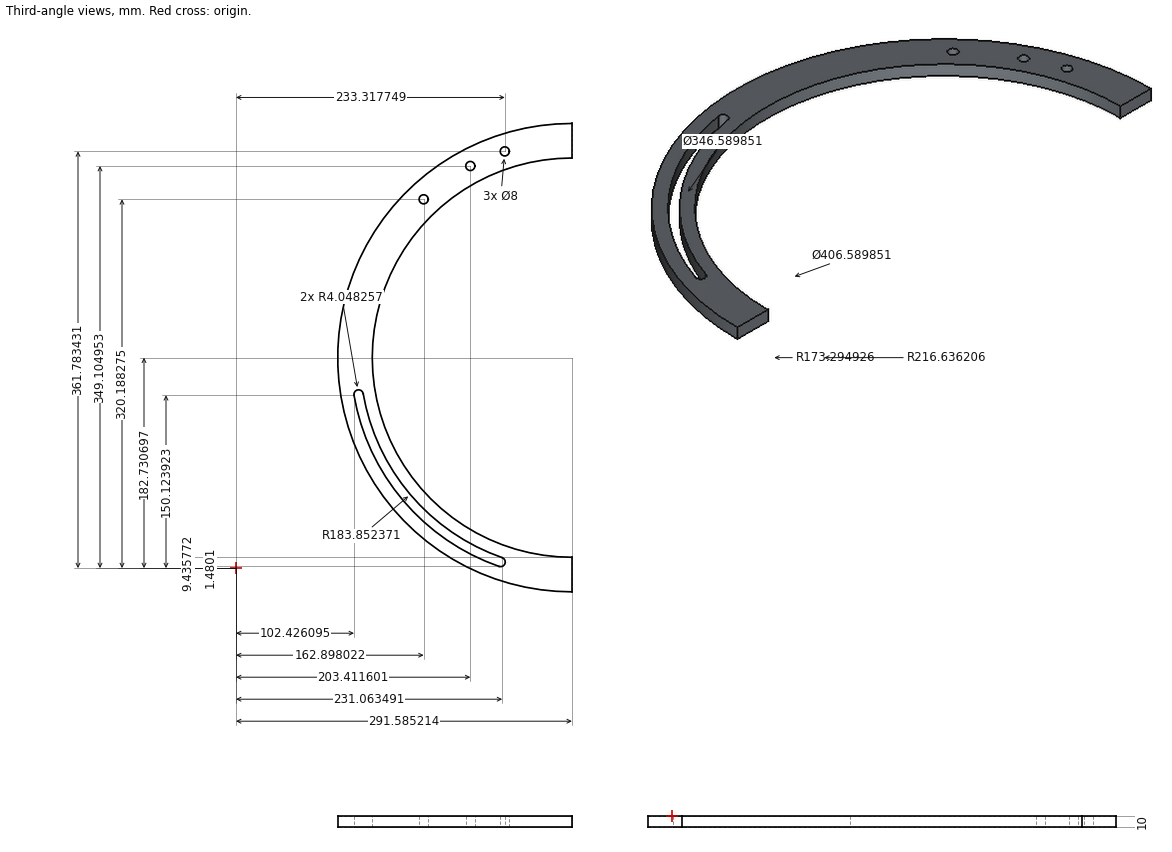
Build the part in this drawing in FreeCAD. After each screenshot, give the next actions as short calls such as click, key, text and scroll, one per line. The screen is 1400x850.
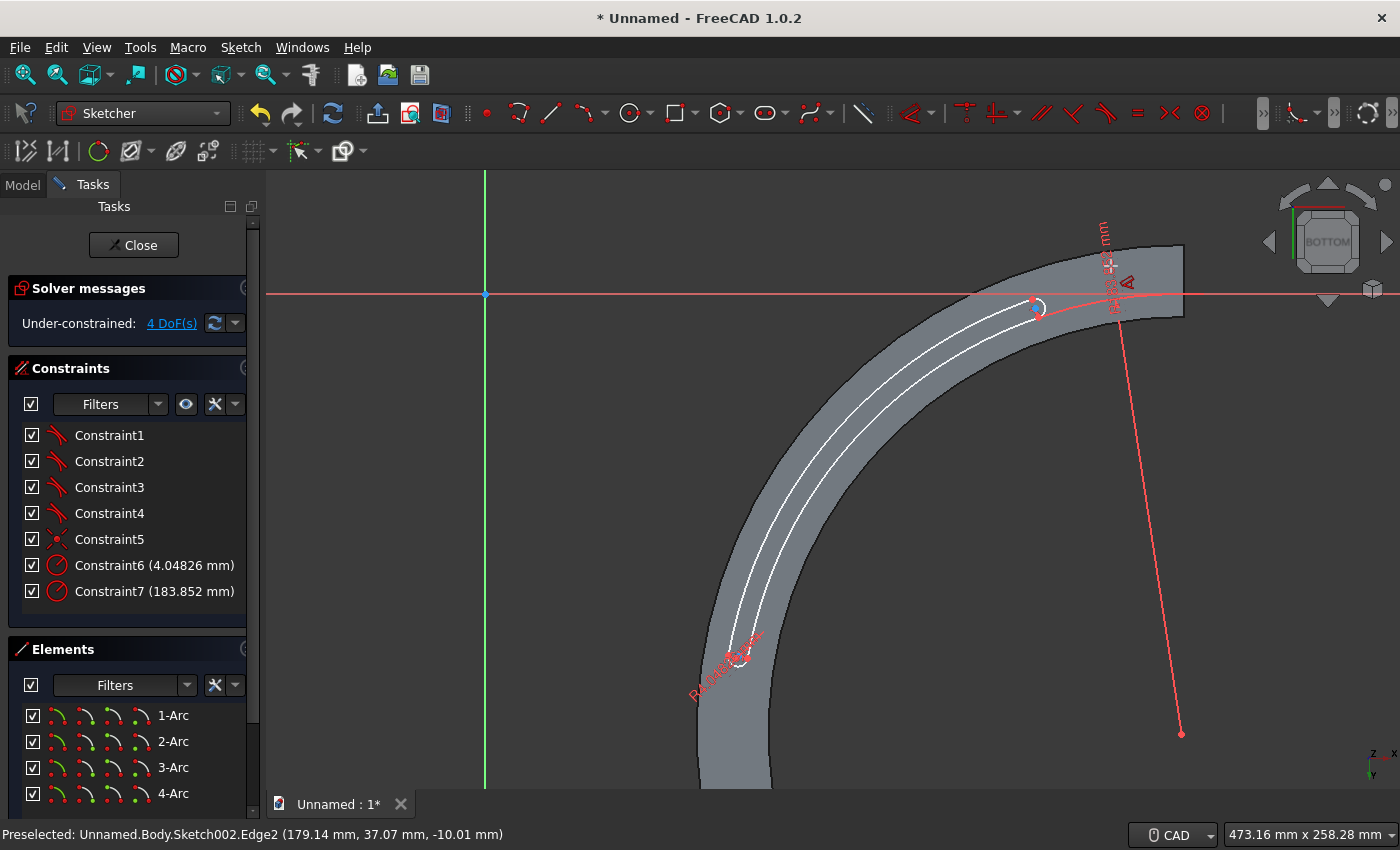
scroll(1032, 299, up, 13)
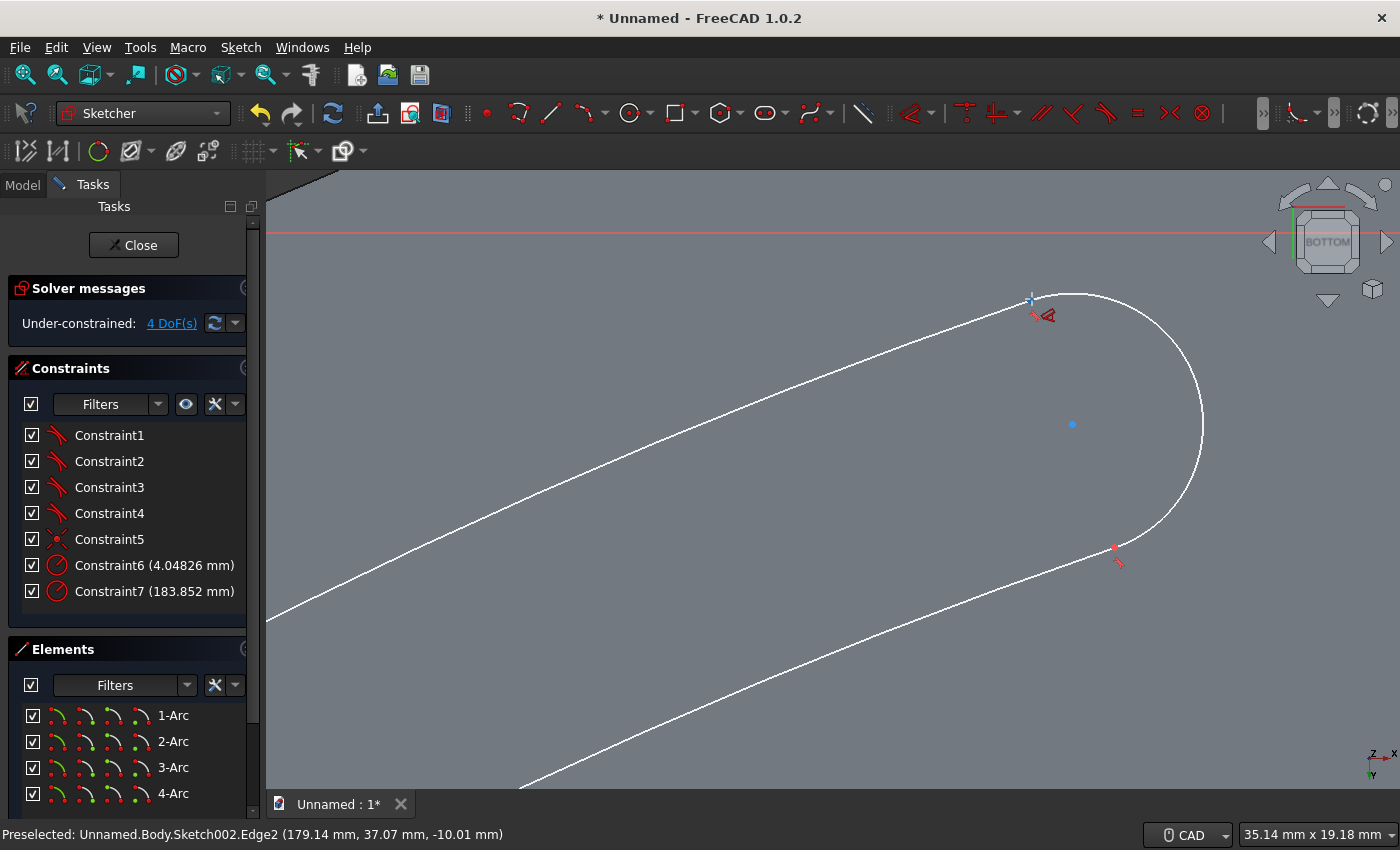
click(1030, 301)
click(1064, 267)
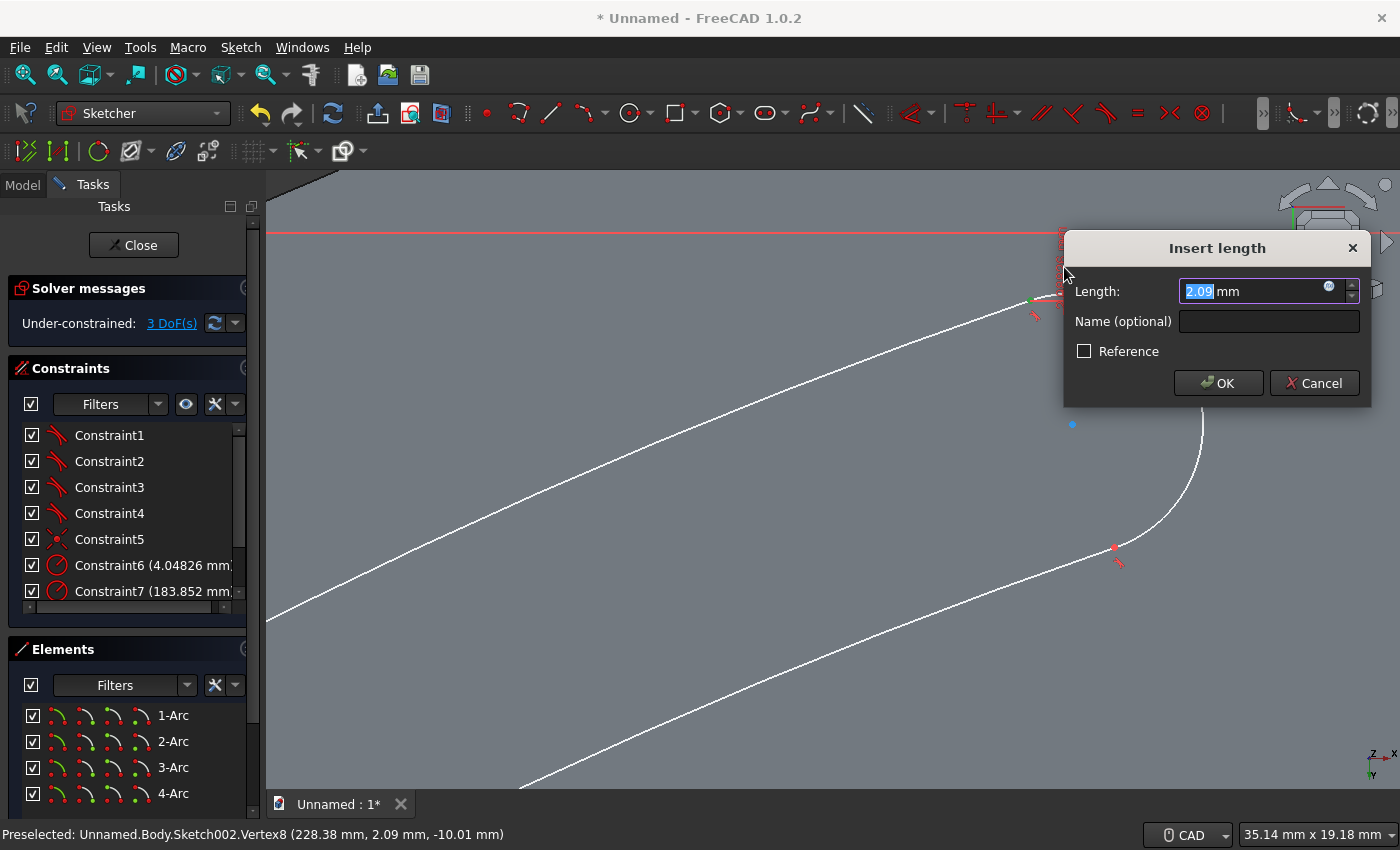
text(1.4801)
key(Return)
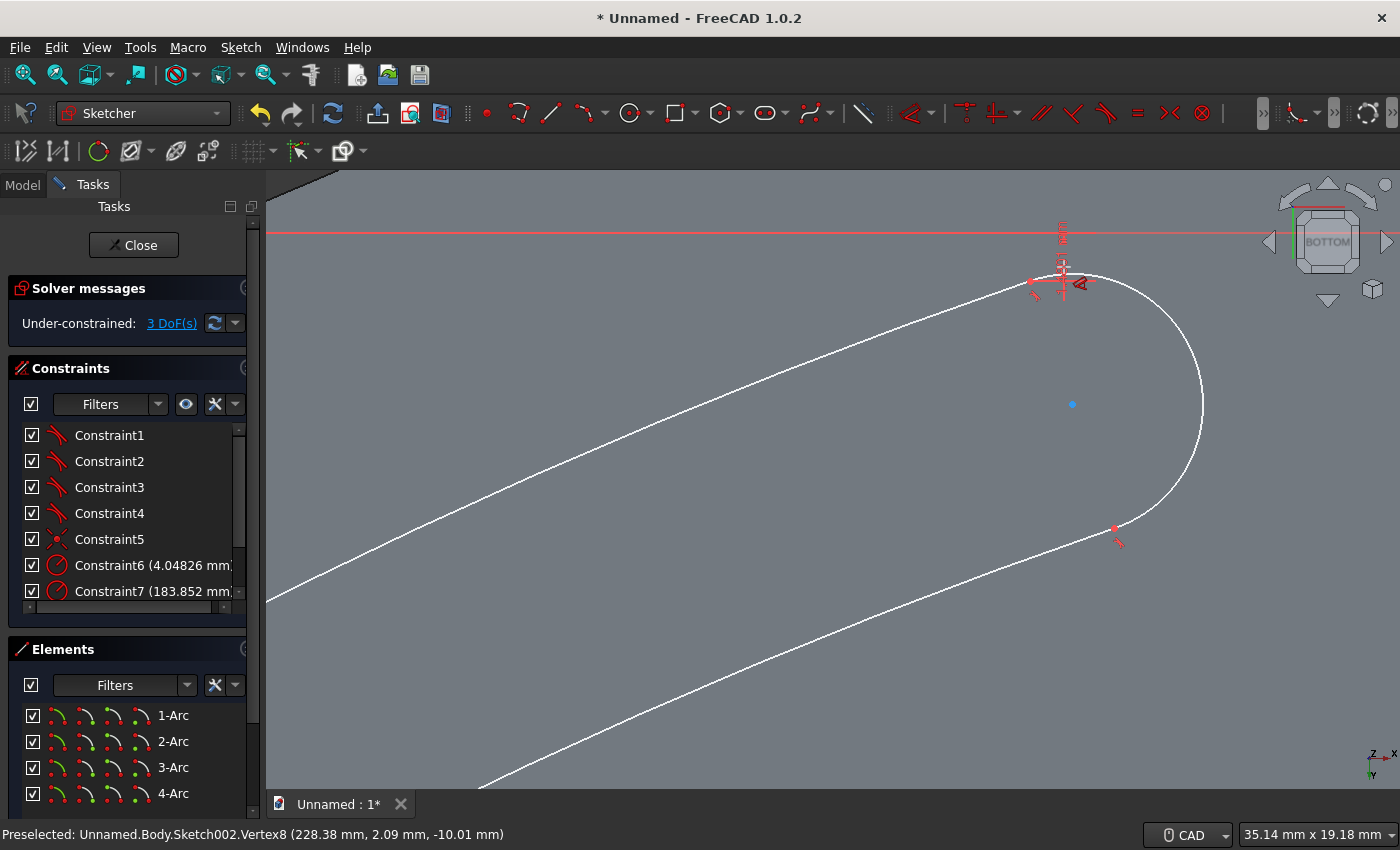
scroll(1032, 299, down, 13)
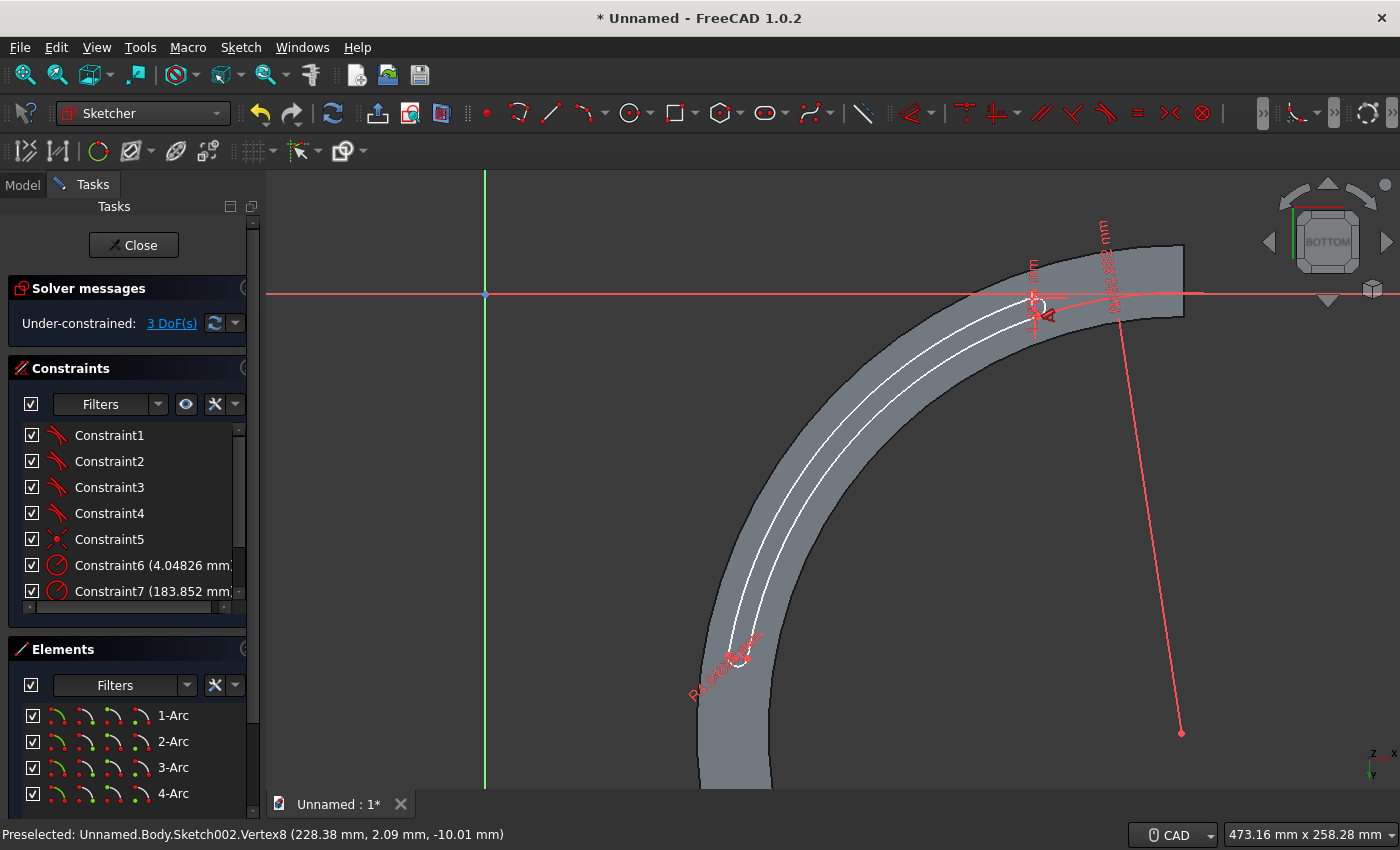
scroll(728, 655, up, 2)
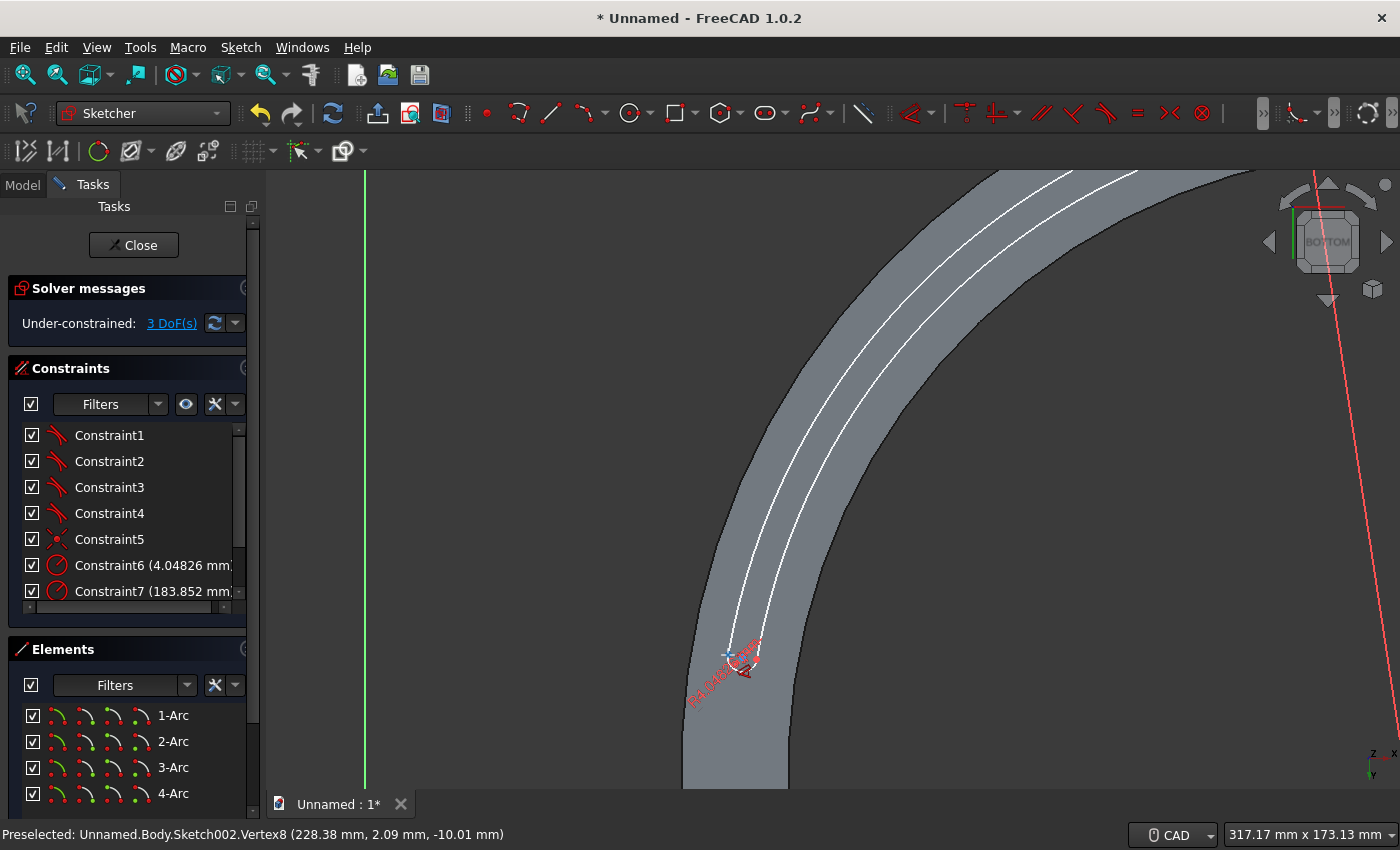
click(728, 655)
click(547, 689)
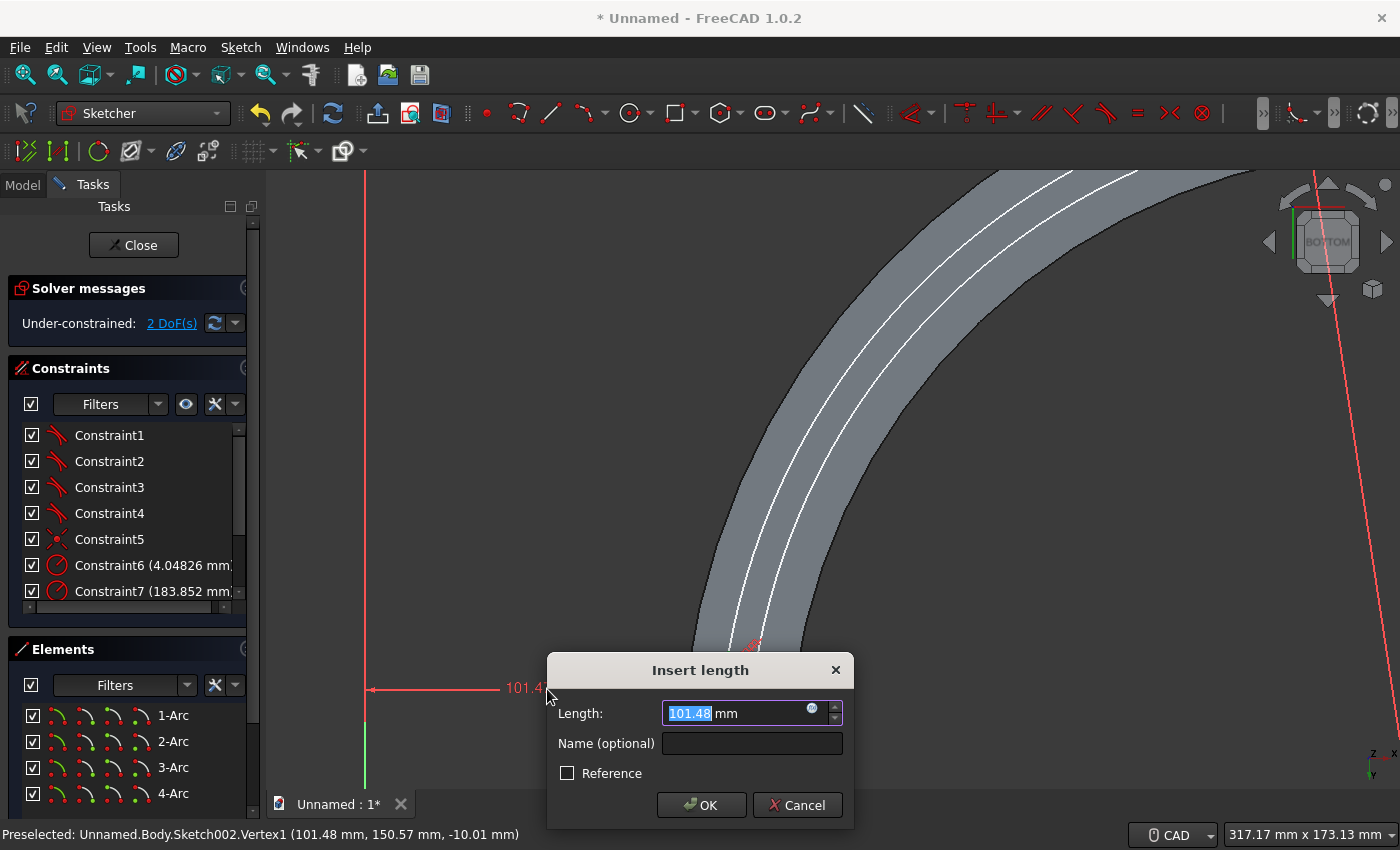
text(102.426095)
key(Return)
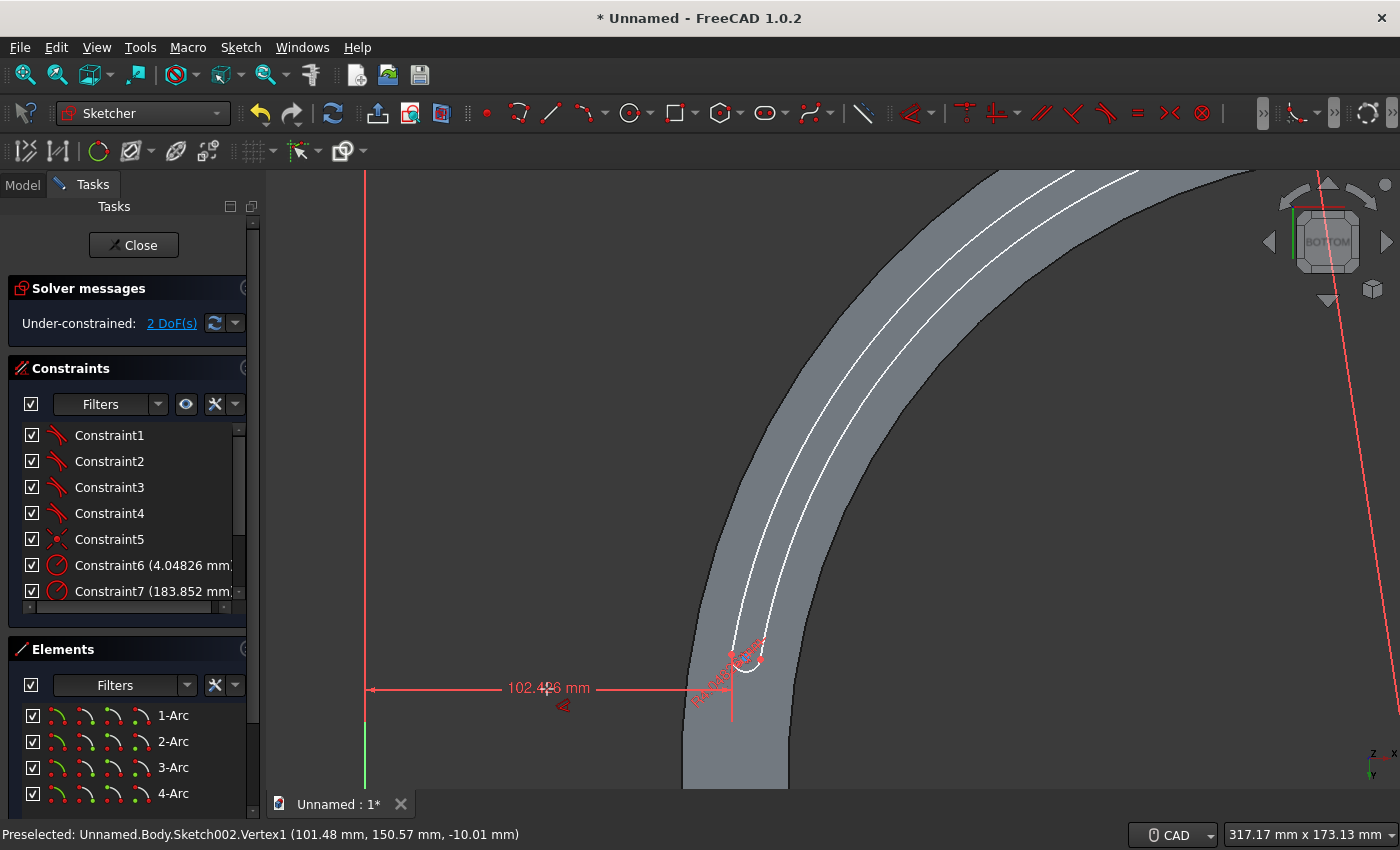
click(732, 655)
click(331, 426)